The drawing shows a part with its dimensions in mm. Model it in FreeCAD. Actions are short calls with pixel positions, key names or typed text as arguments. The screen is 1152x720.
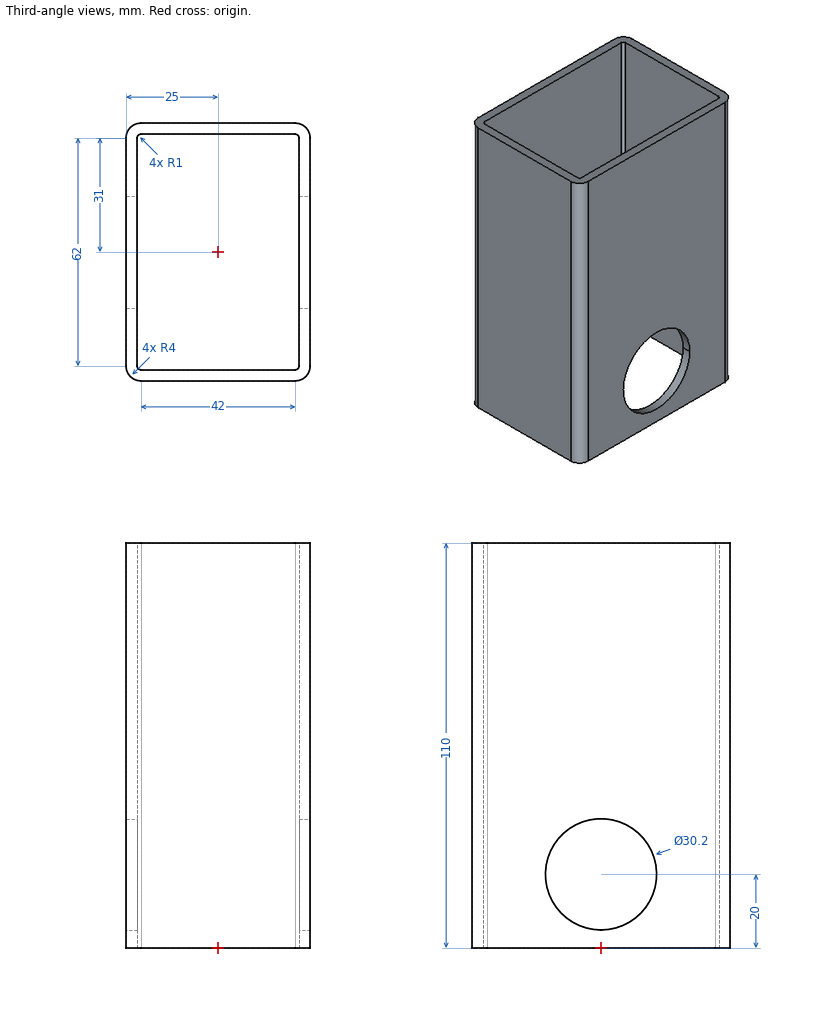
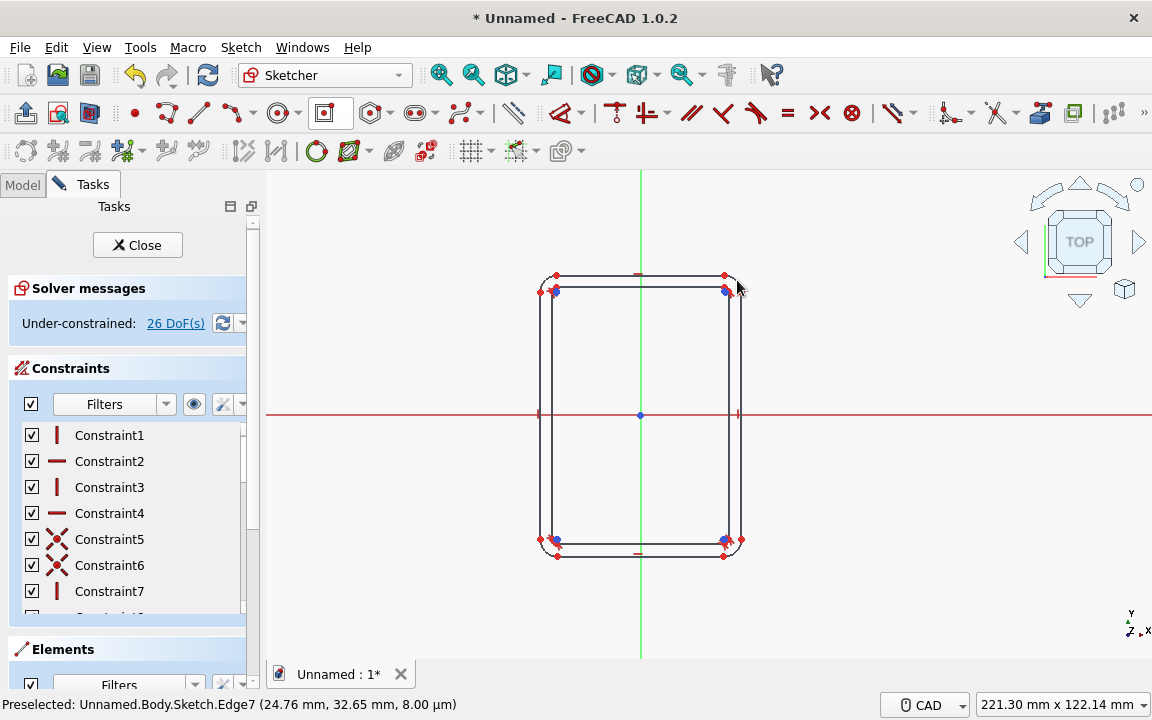
click(674, 276)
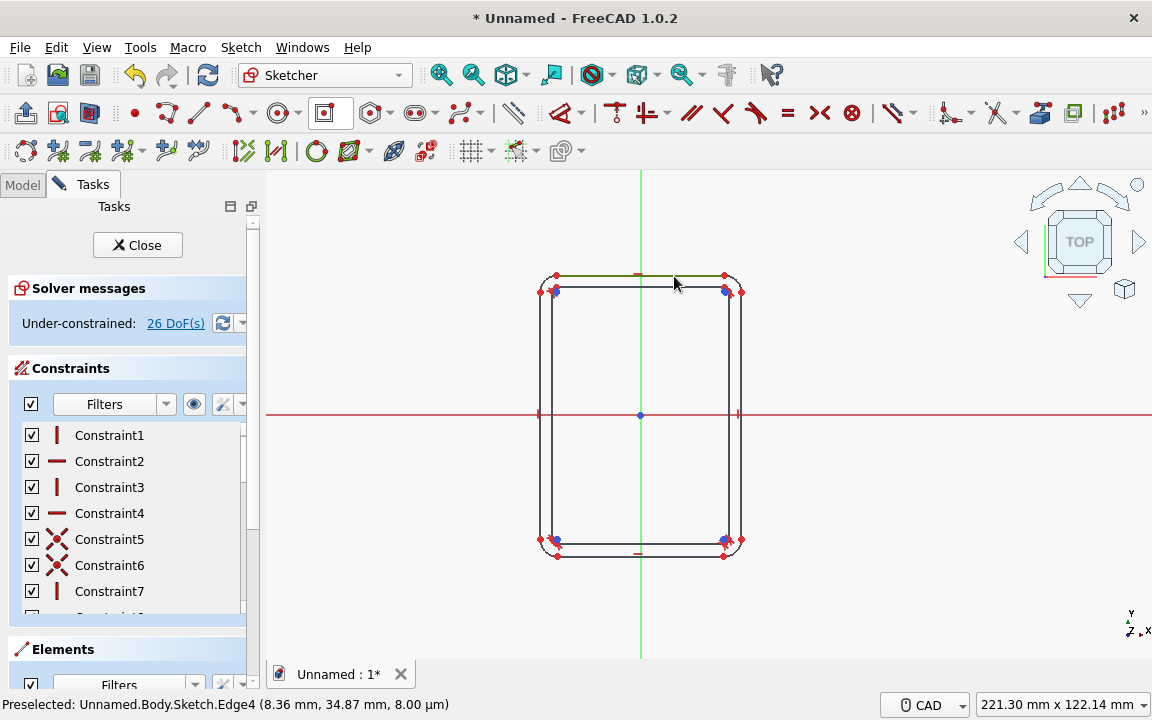
click(737, 281)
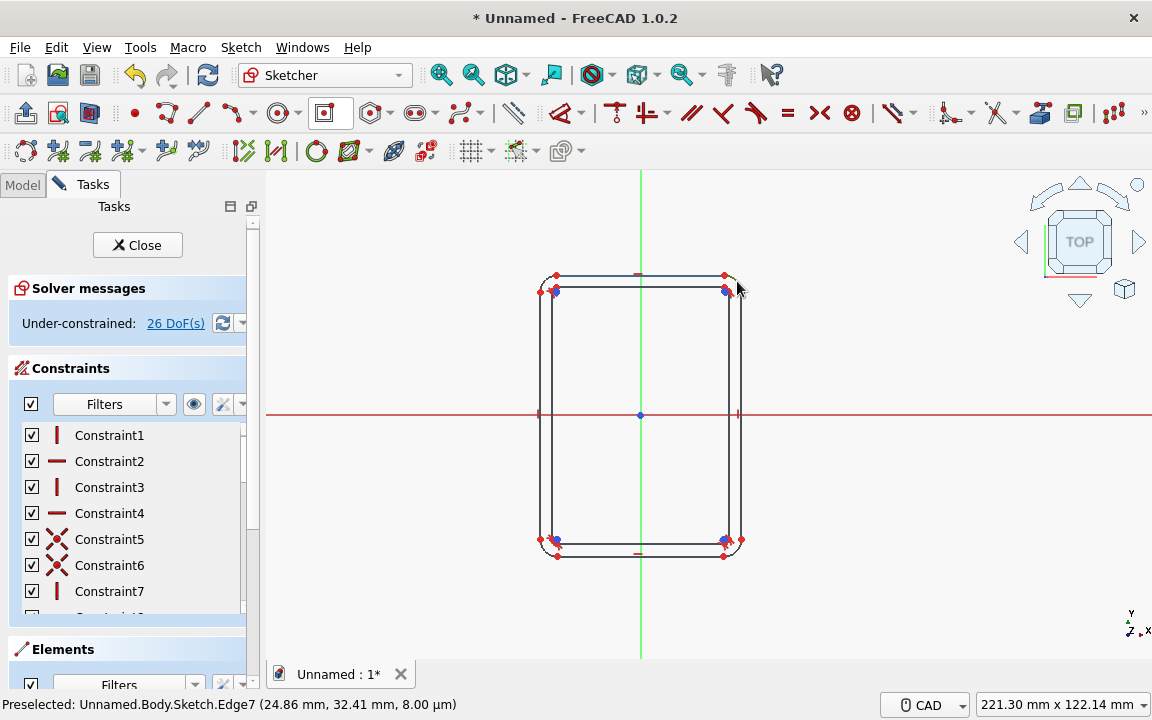
click(756, 114)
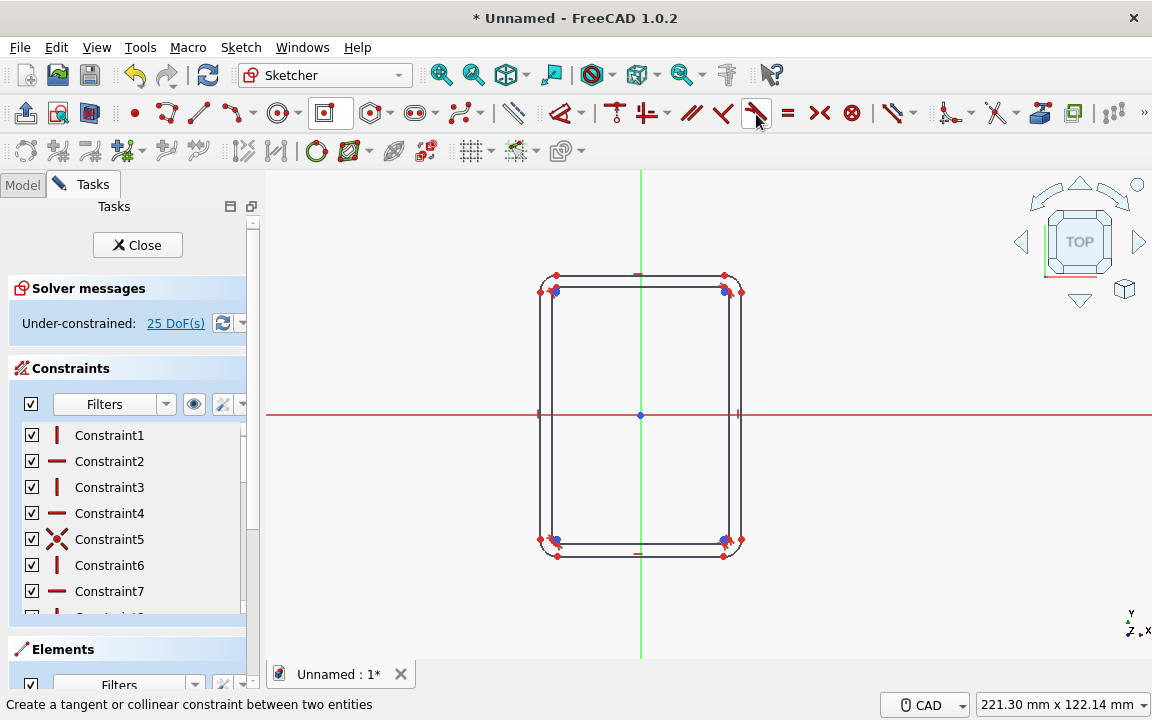
click(674, 276)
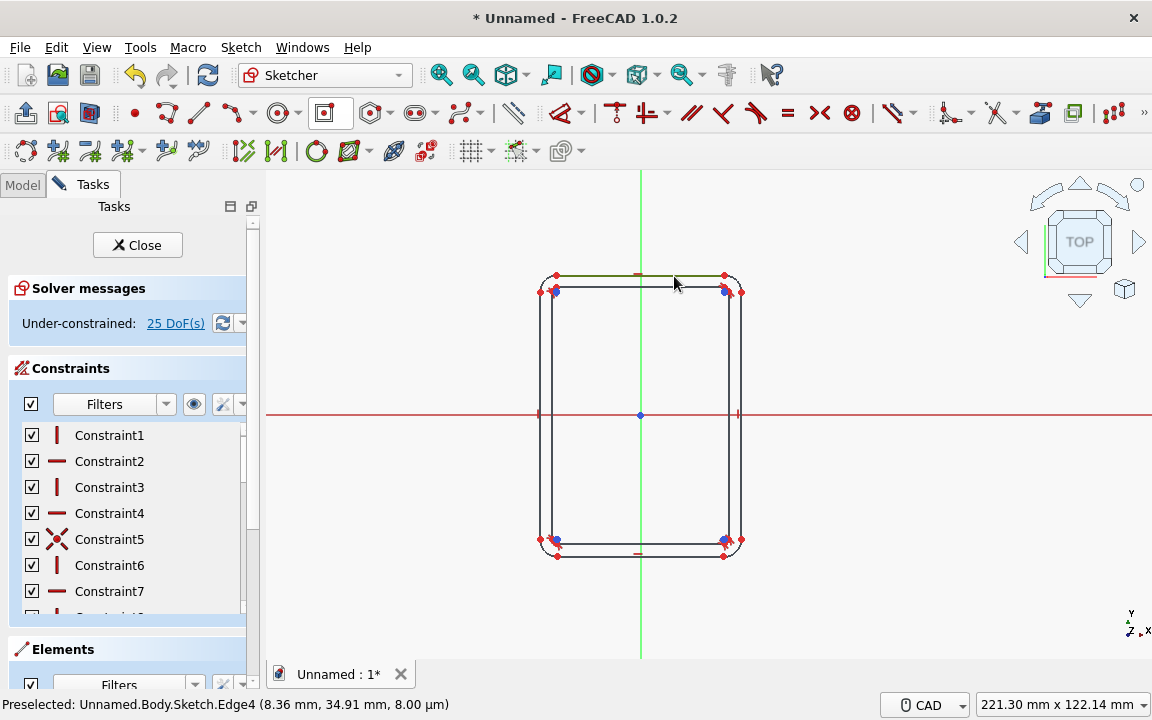
click(545, 281)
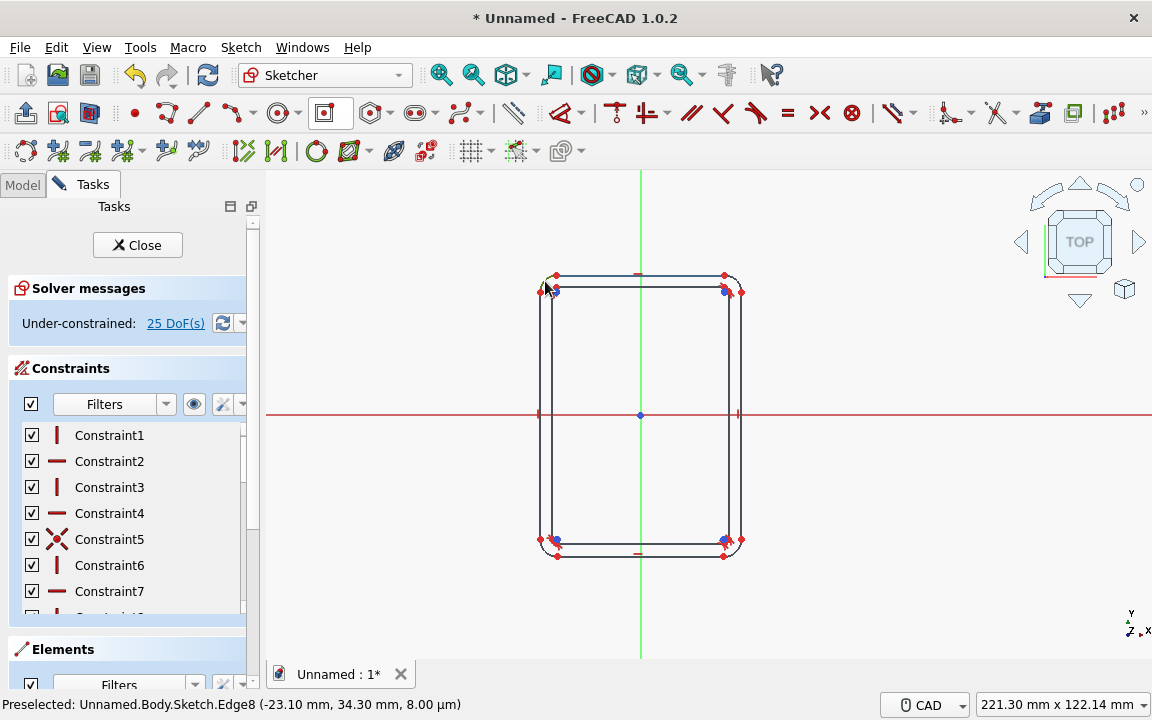
key(t)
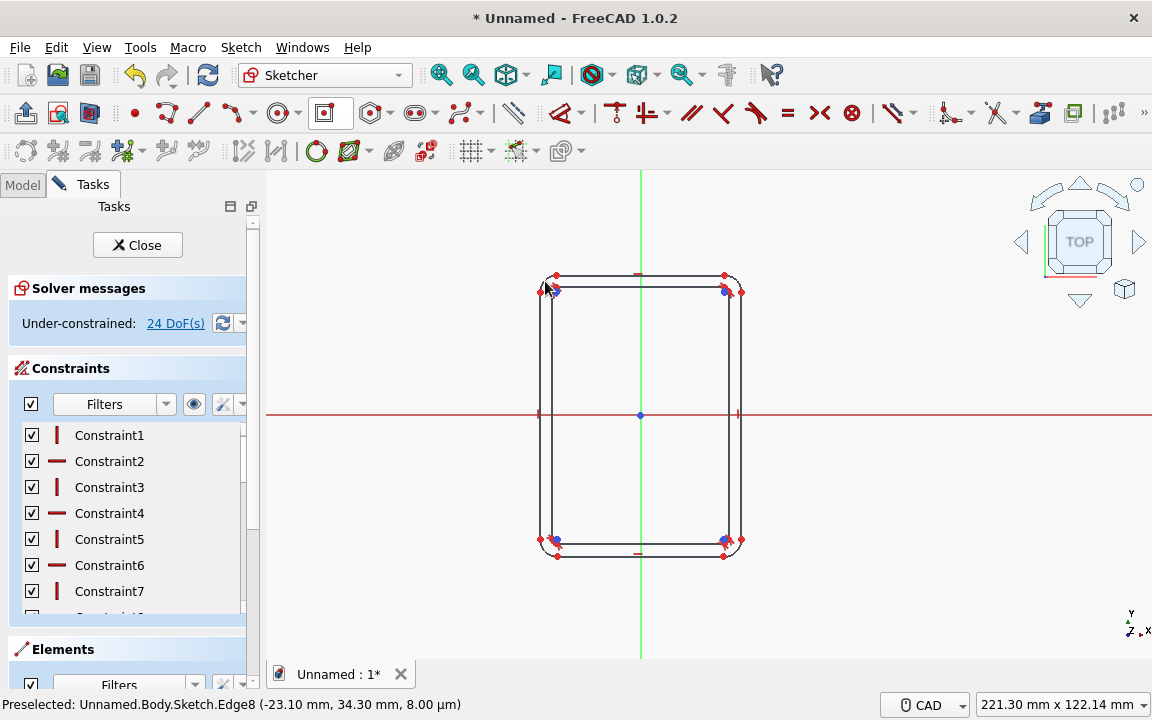
click(552, 465)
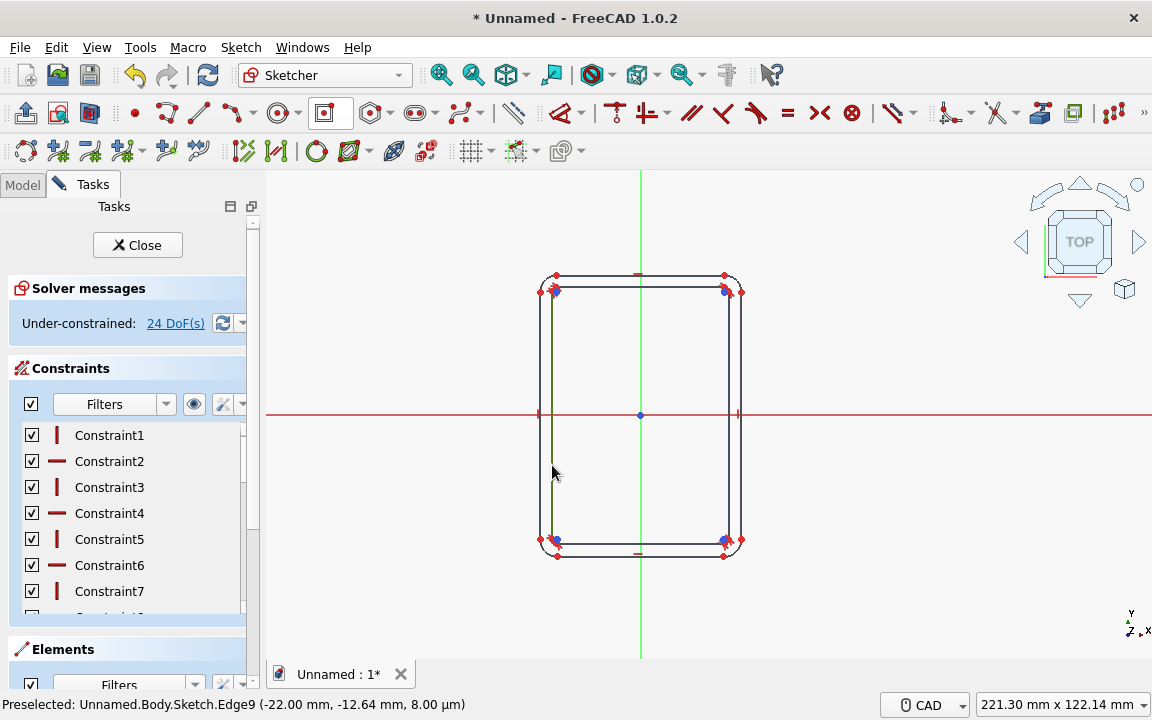
scroll(553, 289, up, 8)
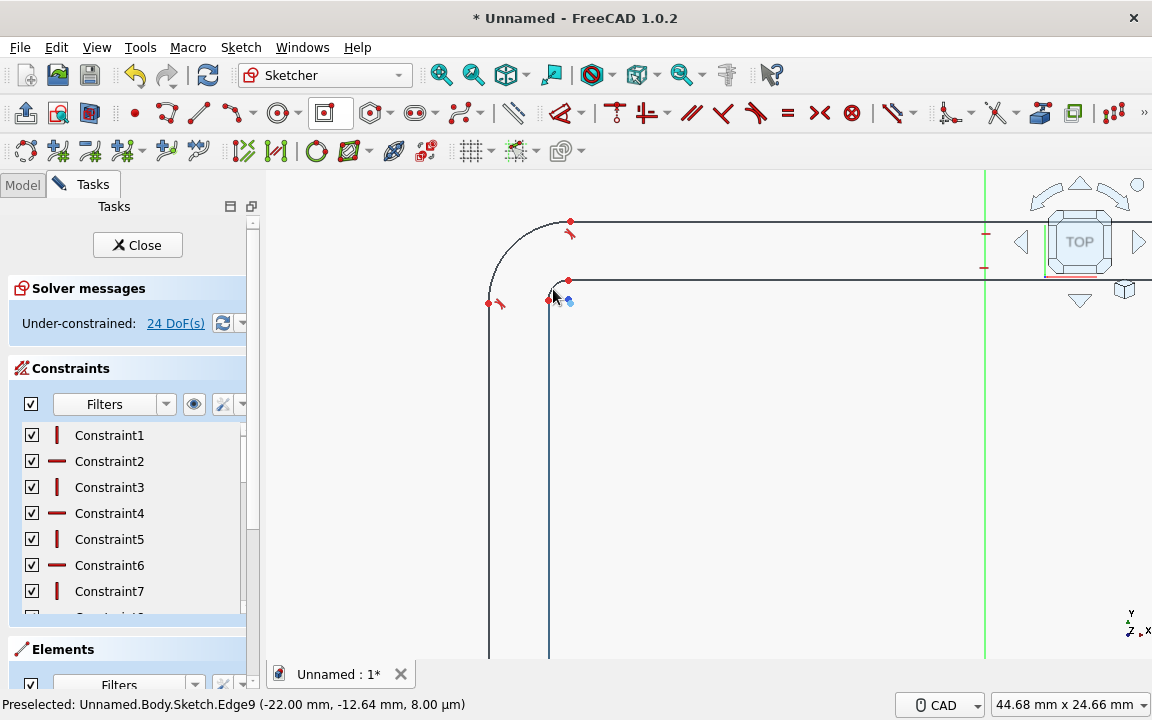
click(554, 286)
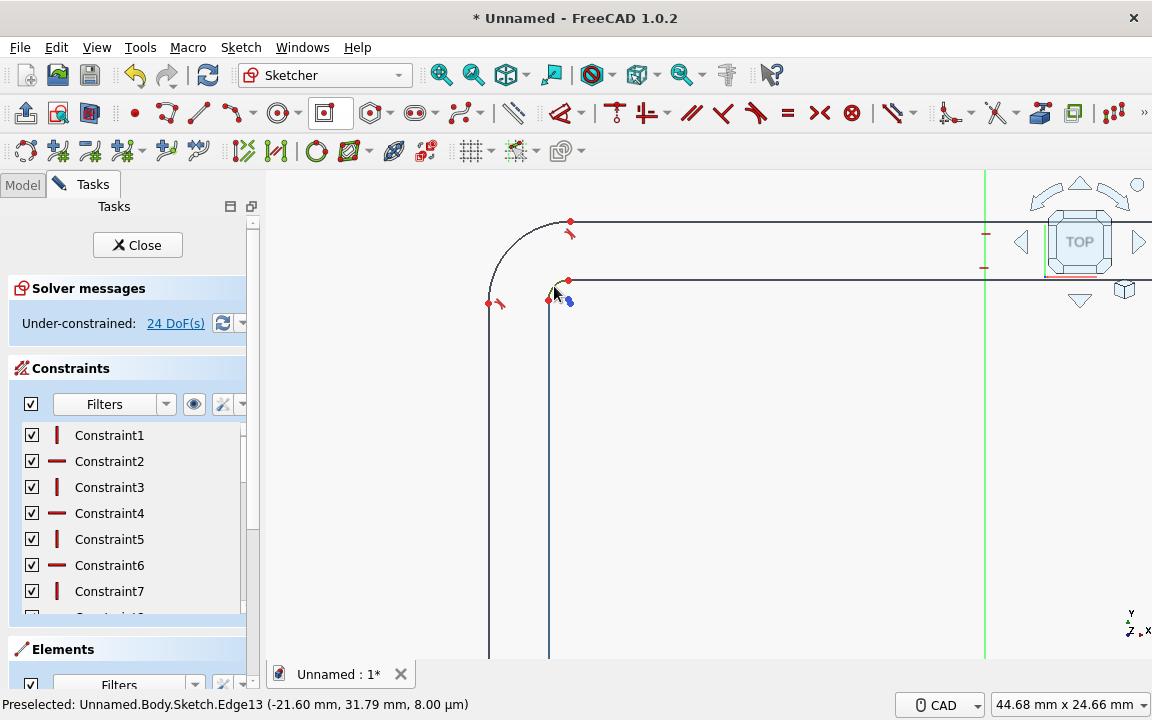
key(t)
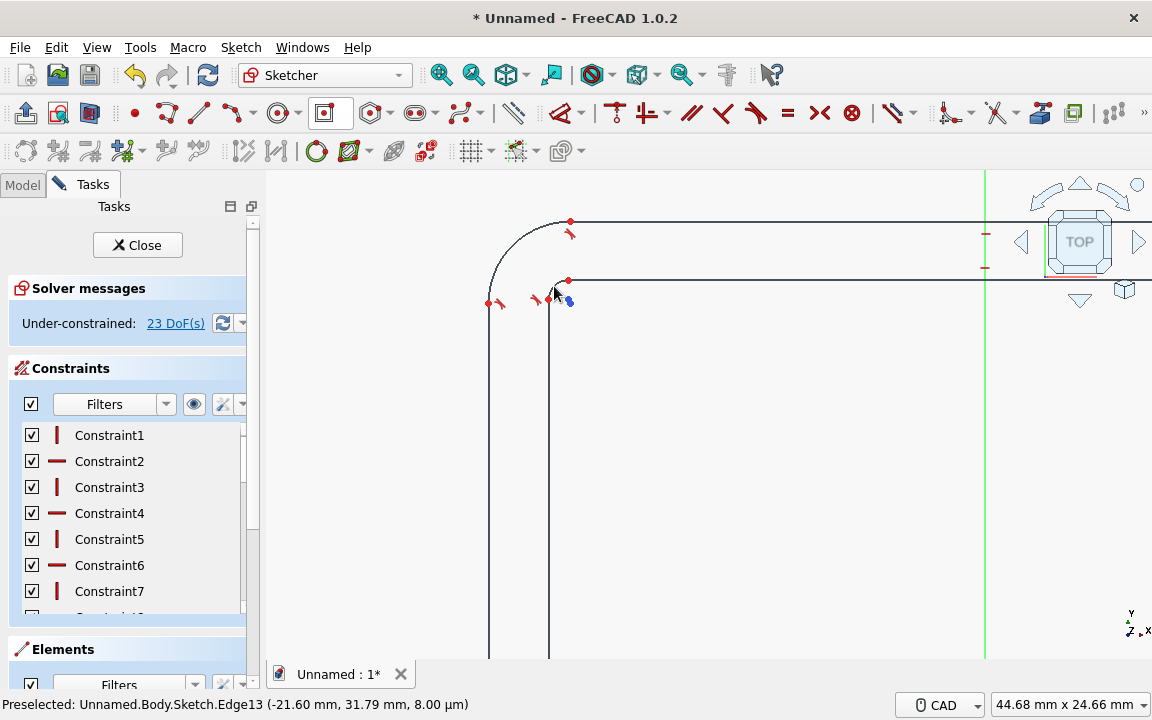
scroll(553, 288, down, 8)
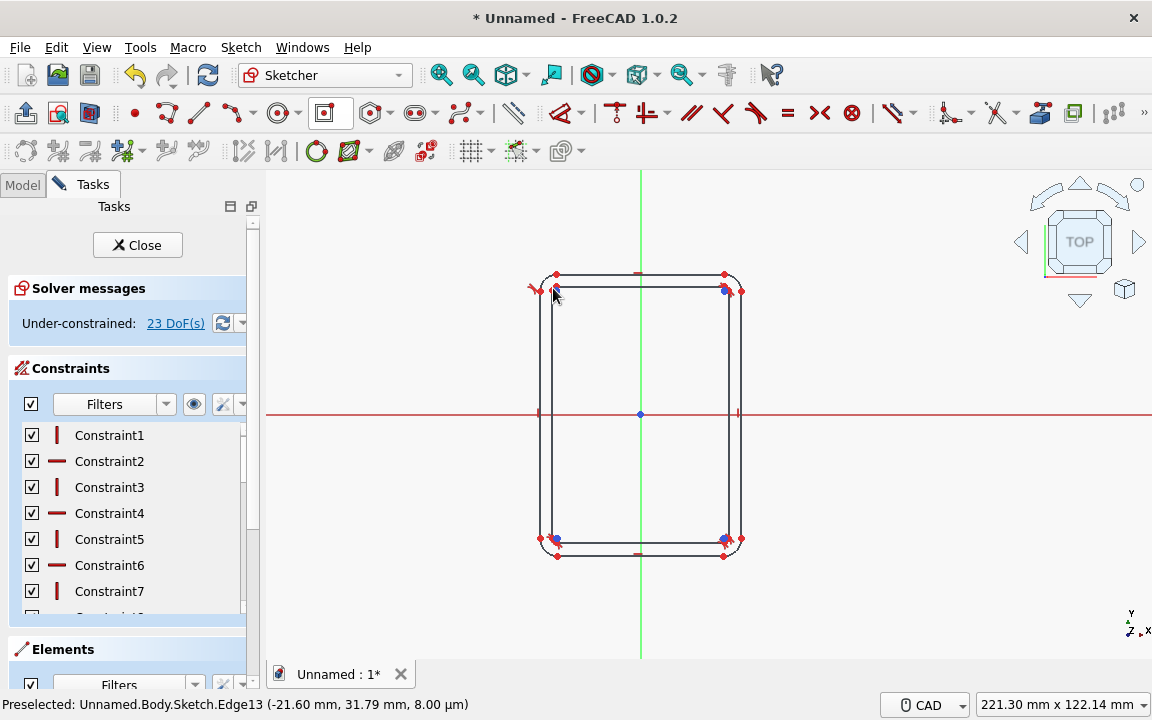
click(552, 340)